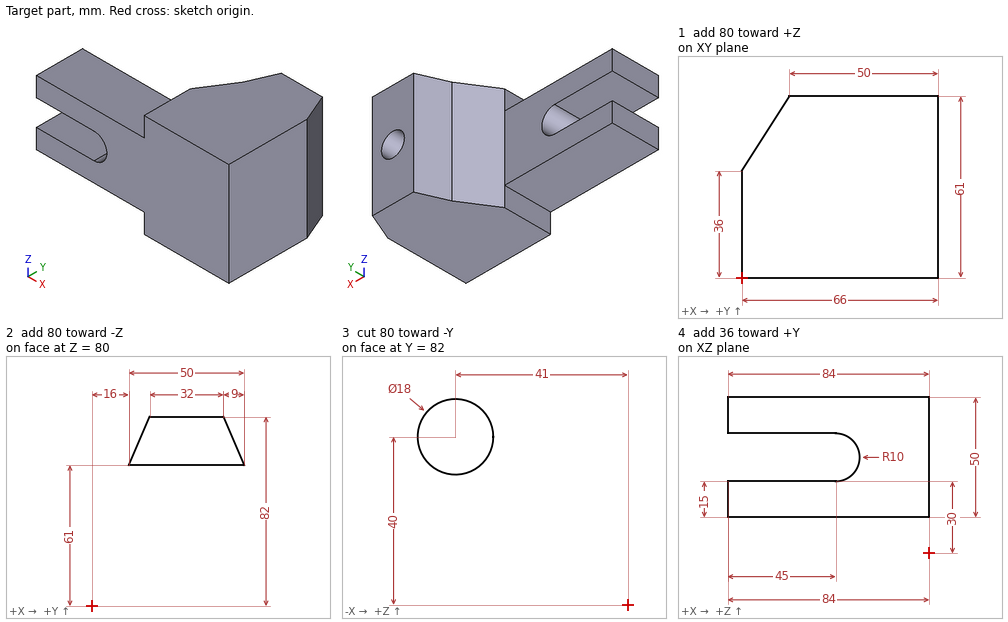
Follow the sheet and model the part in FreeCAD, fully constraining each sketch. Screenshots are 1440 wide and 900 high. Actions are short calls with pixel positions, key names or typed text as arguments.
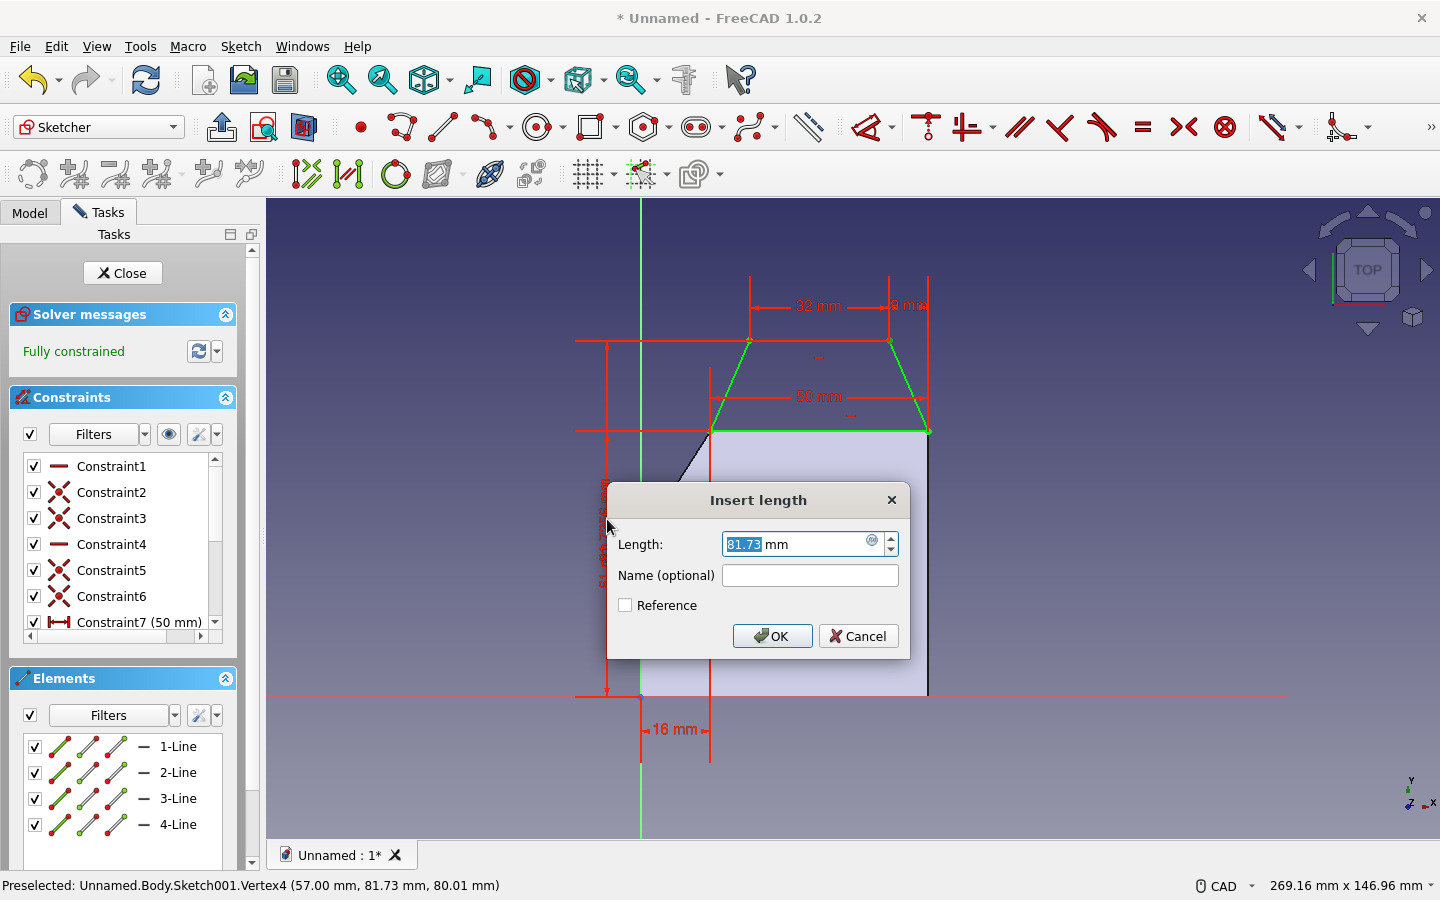
text(82)
key(Return)
key(Escape)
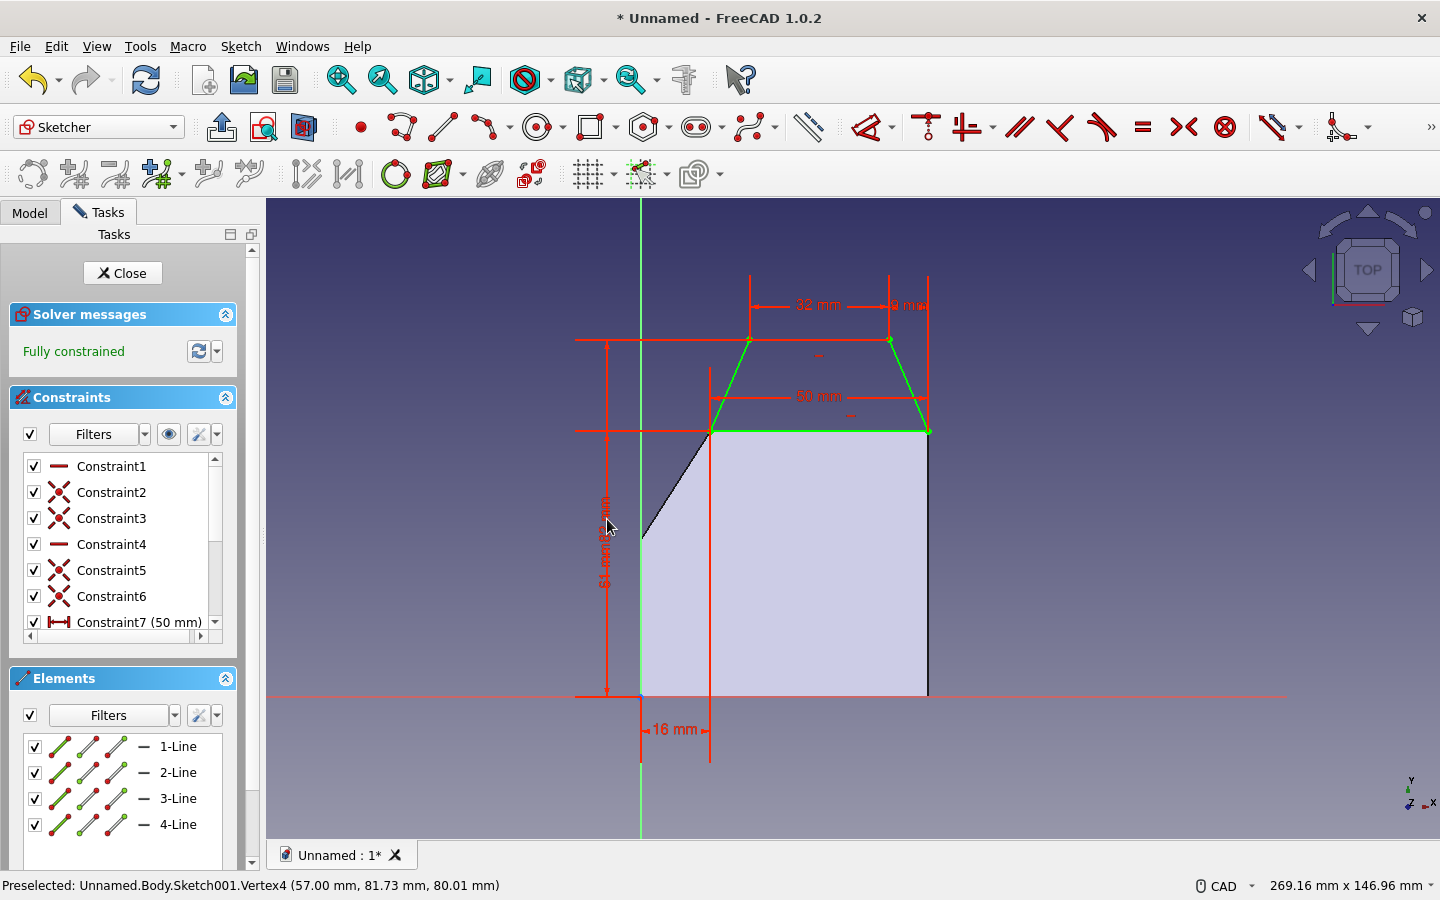
click(123, 273)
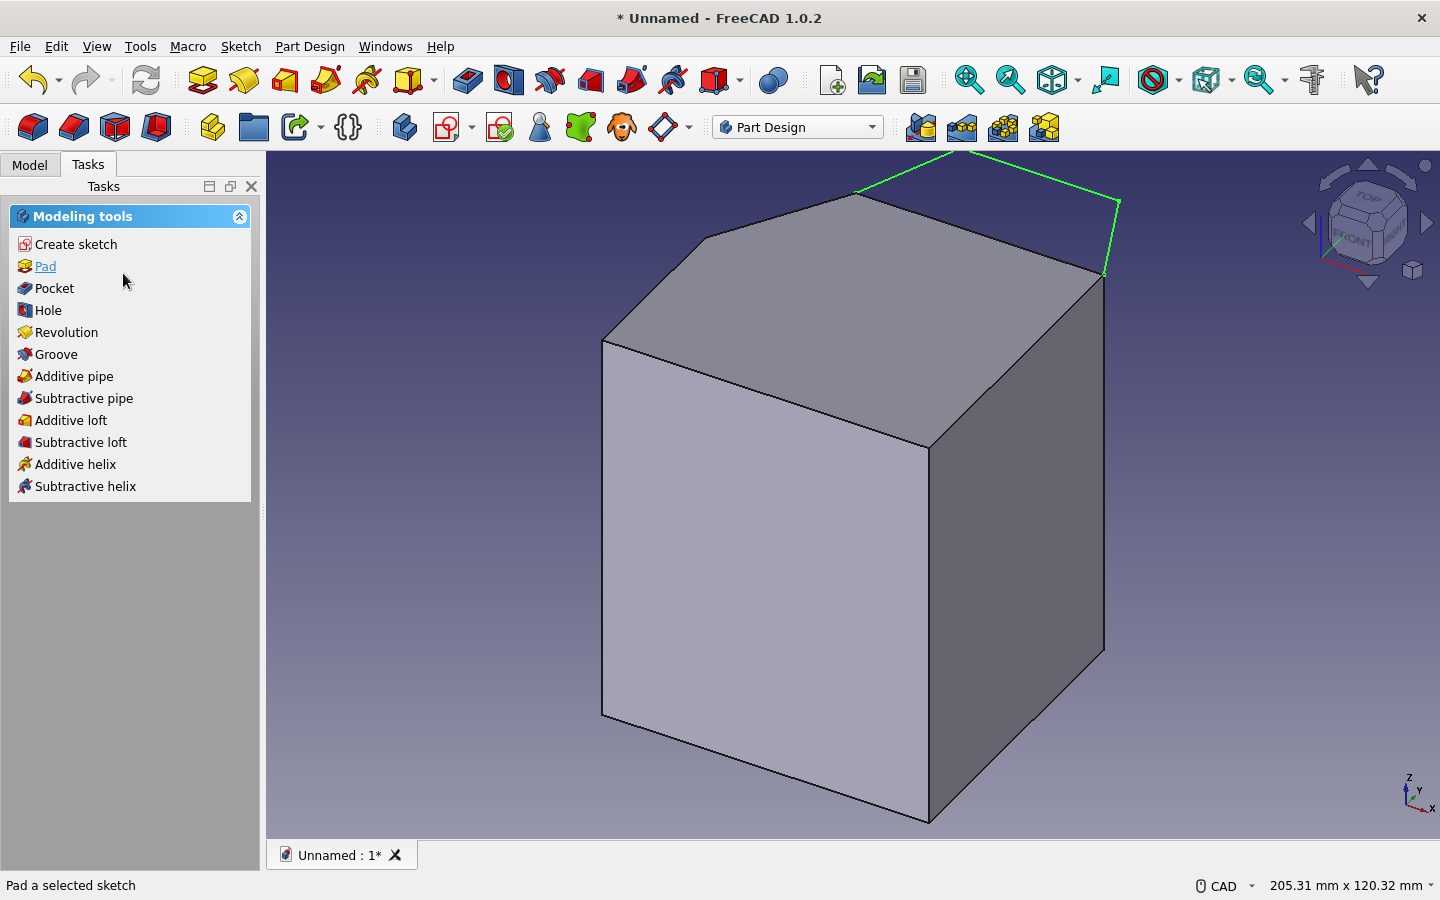
click(203, 80)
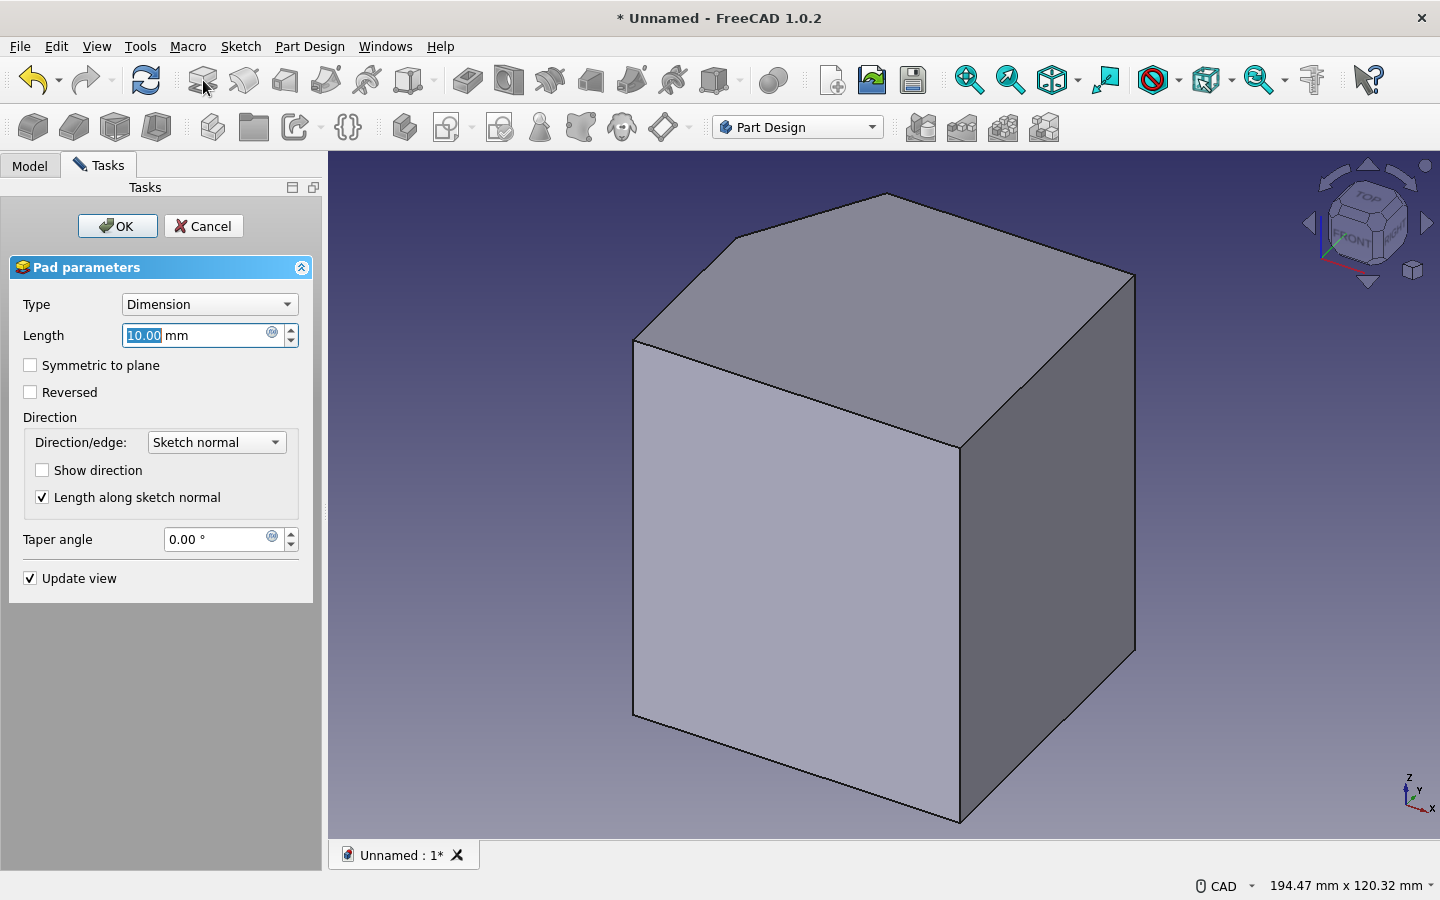
text(80)
key(Tab)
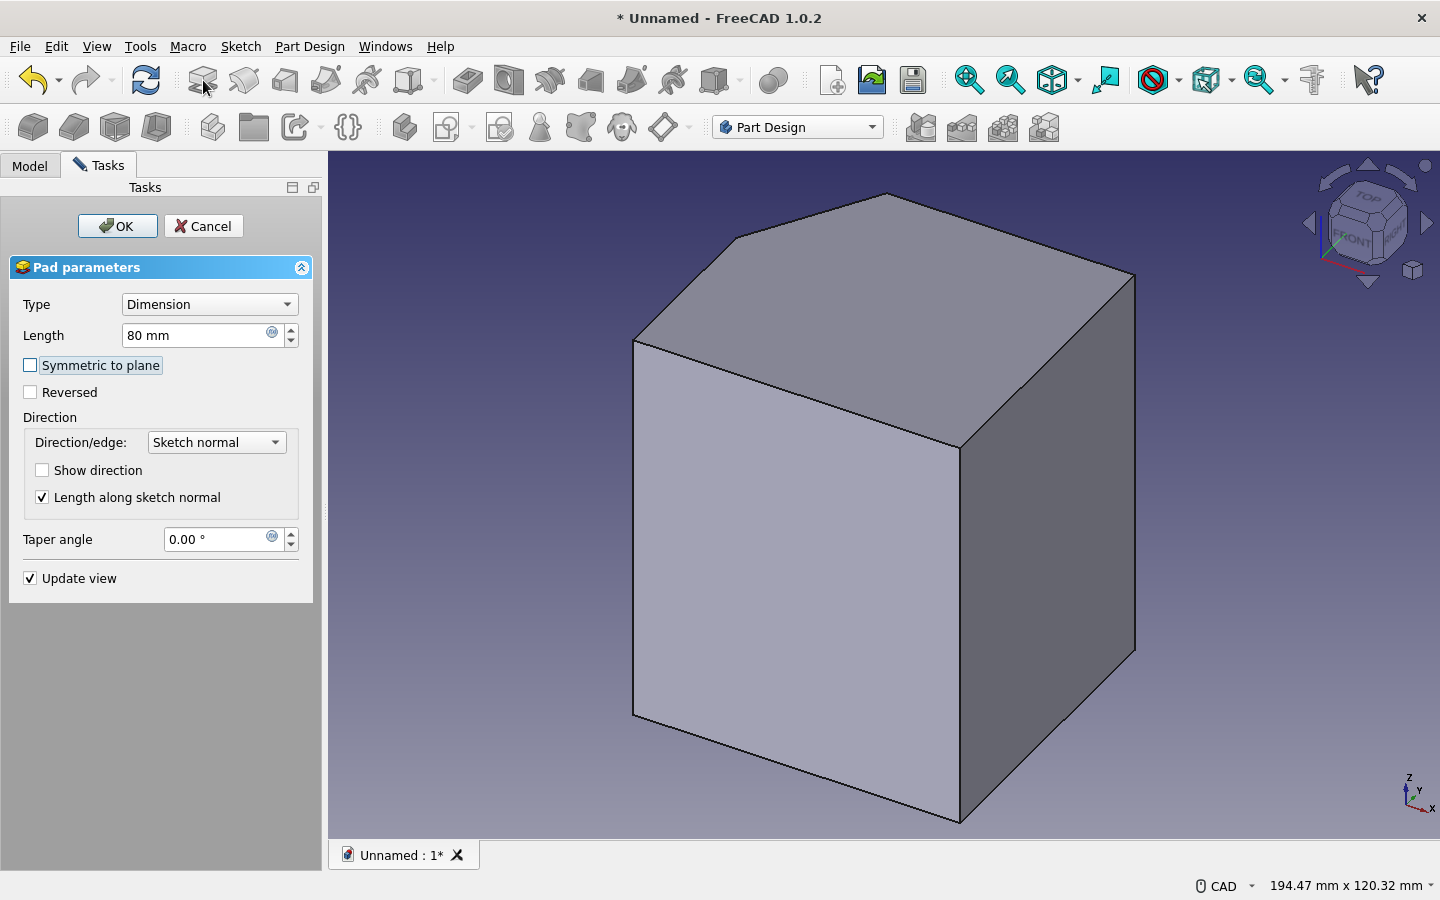
click(31, 392)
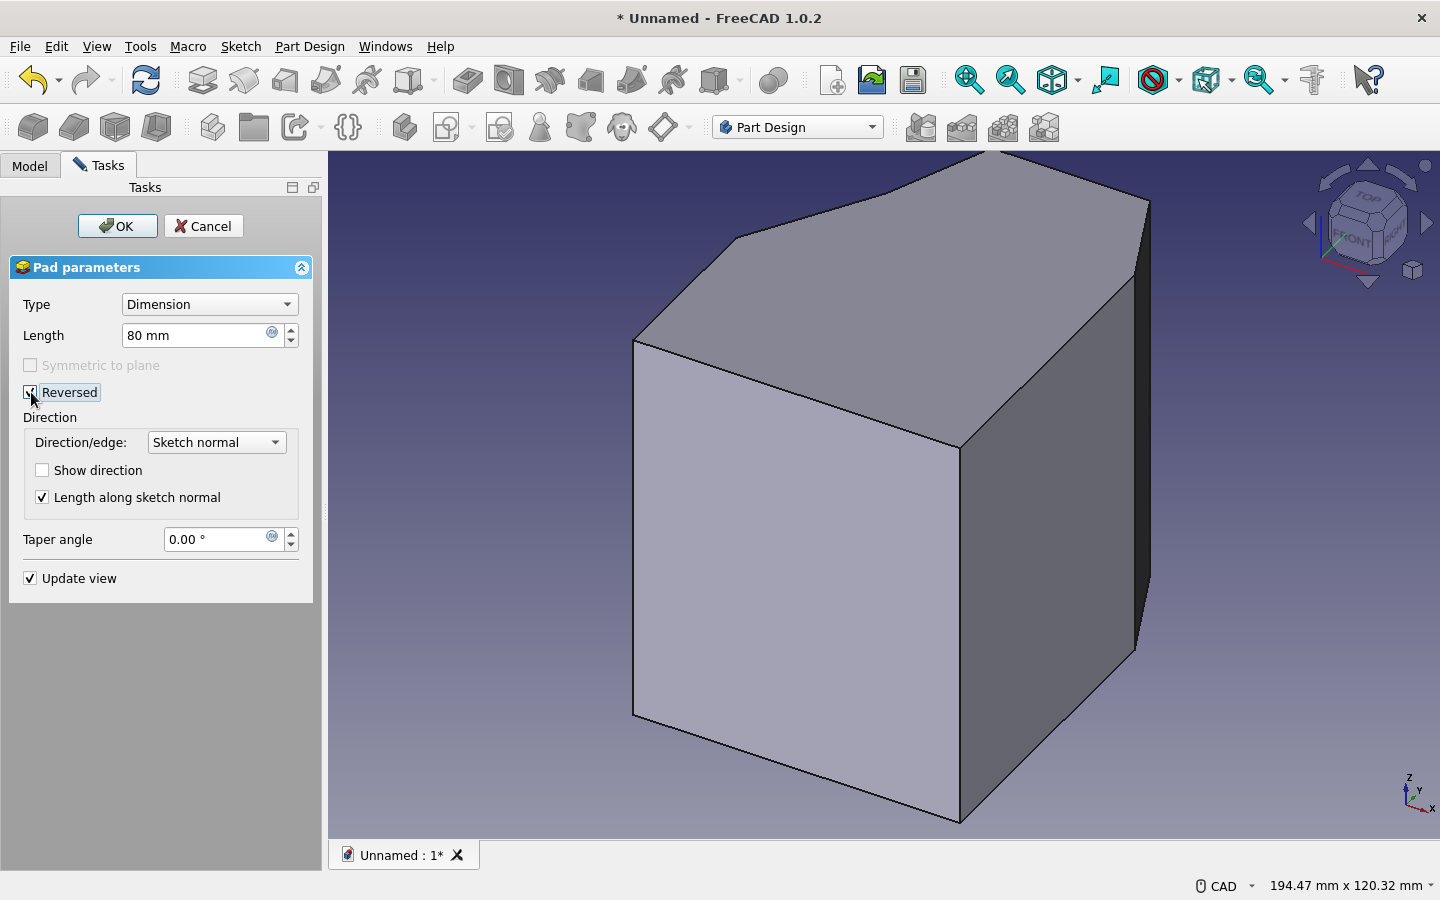
click(118, 226)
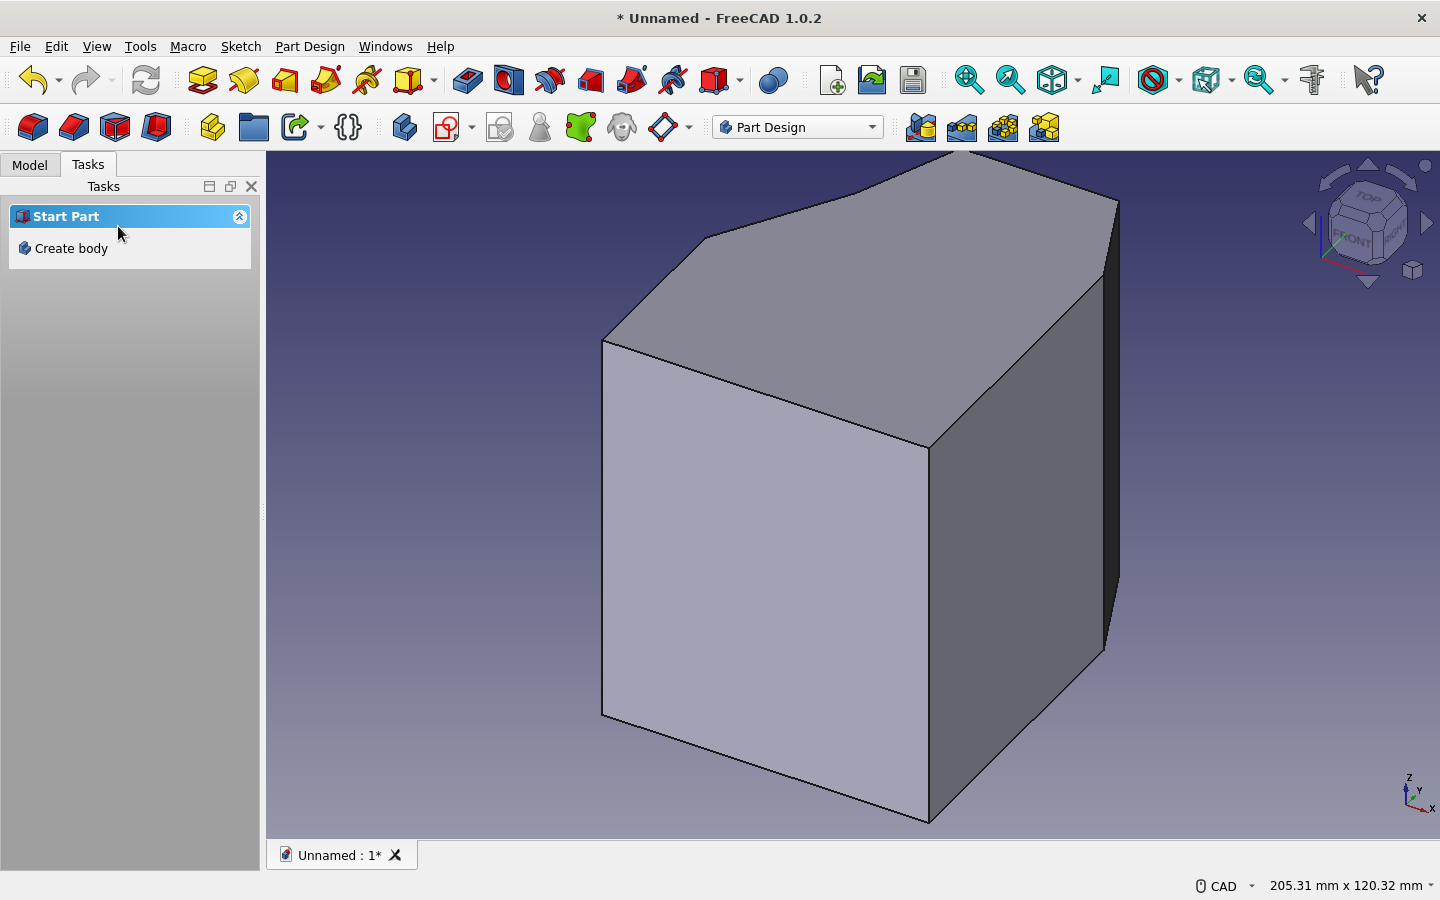
click(970, 80)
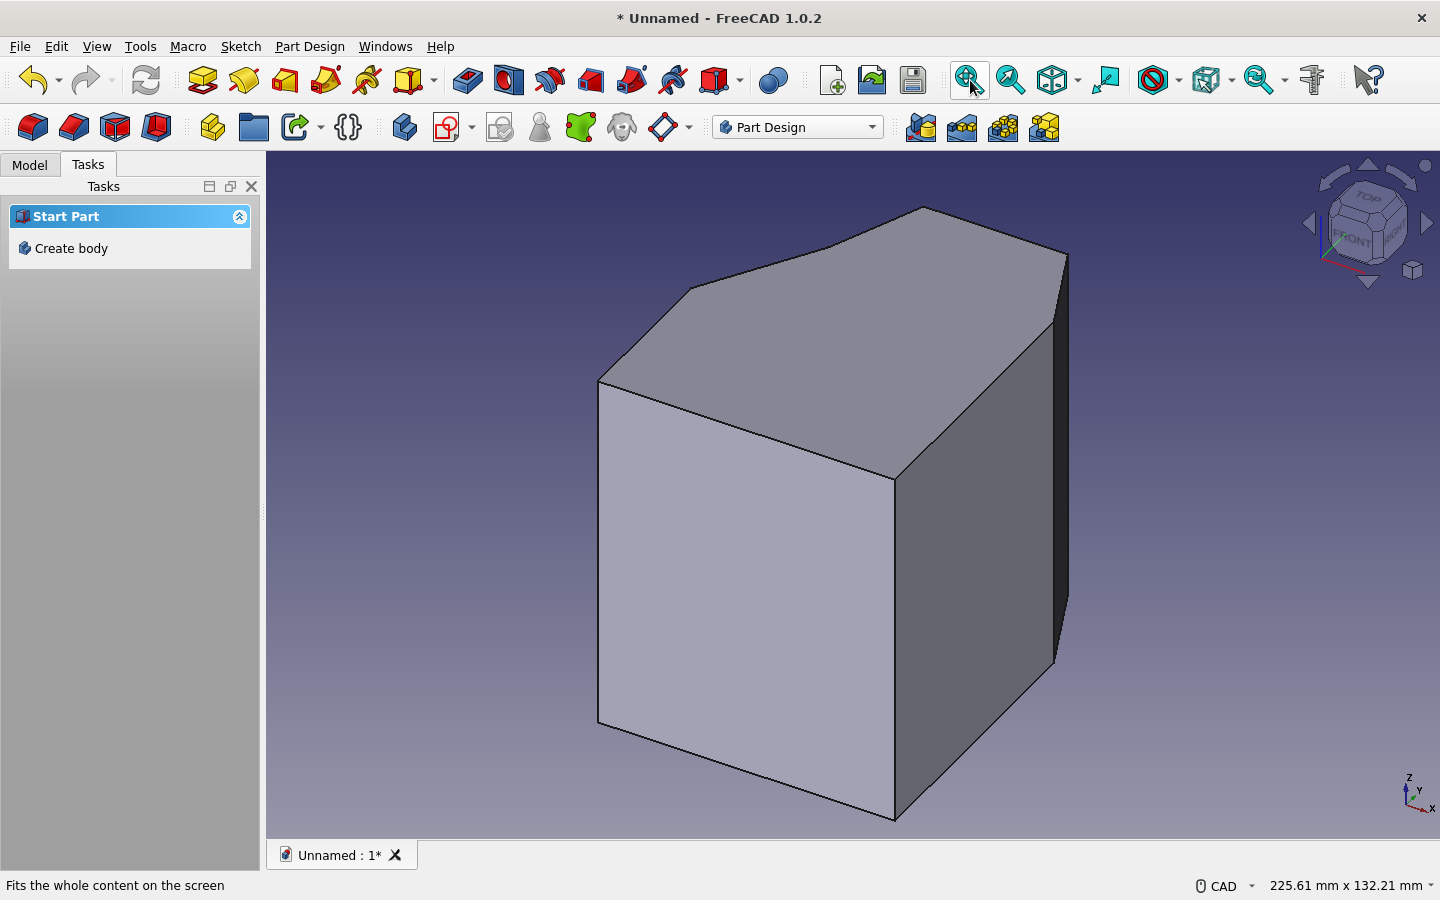
key(4)